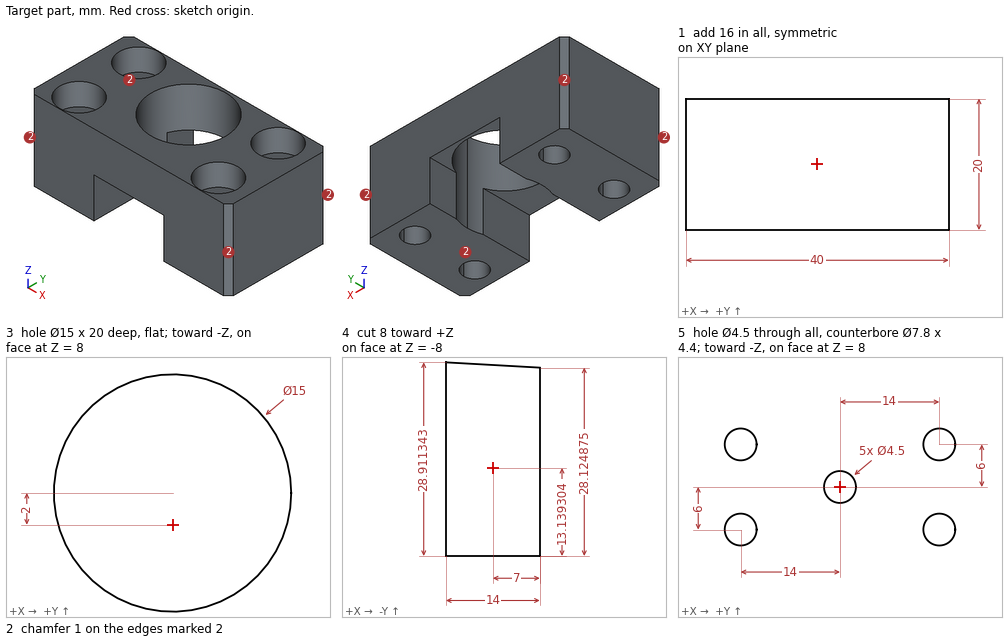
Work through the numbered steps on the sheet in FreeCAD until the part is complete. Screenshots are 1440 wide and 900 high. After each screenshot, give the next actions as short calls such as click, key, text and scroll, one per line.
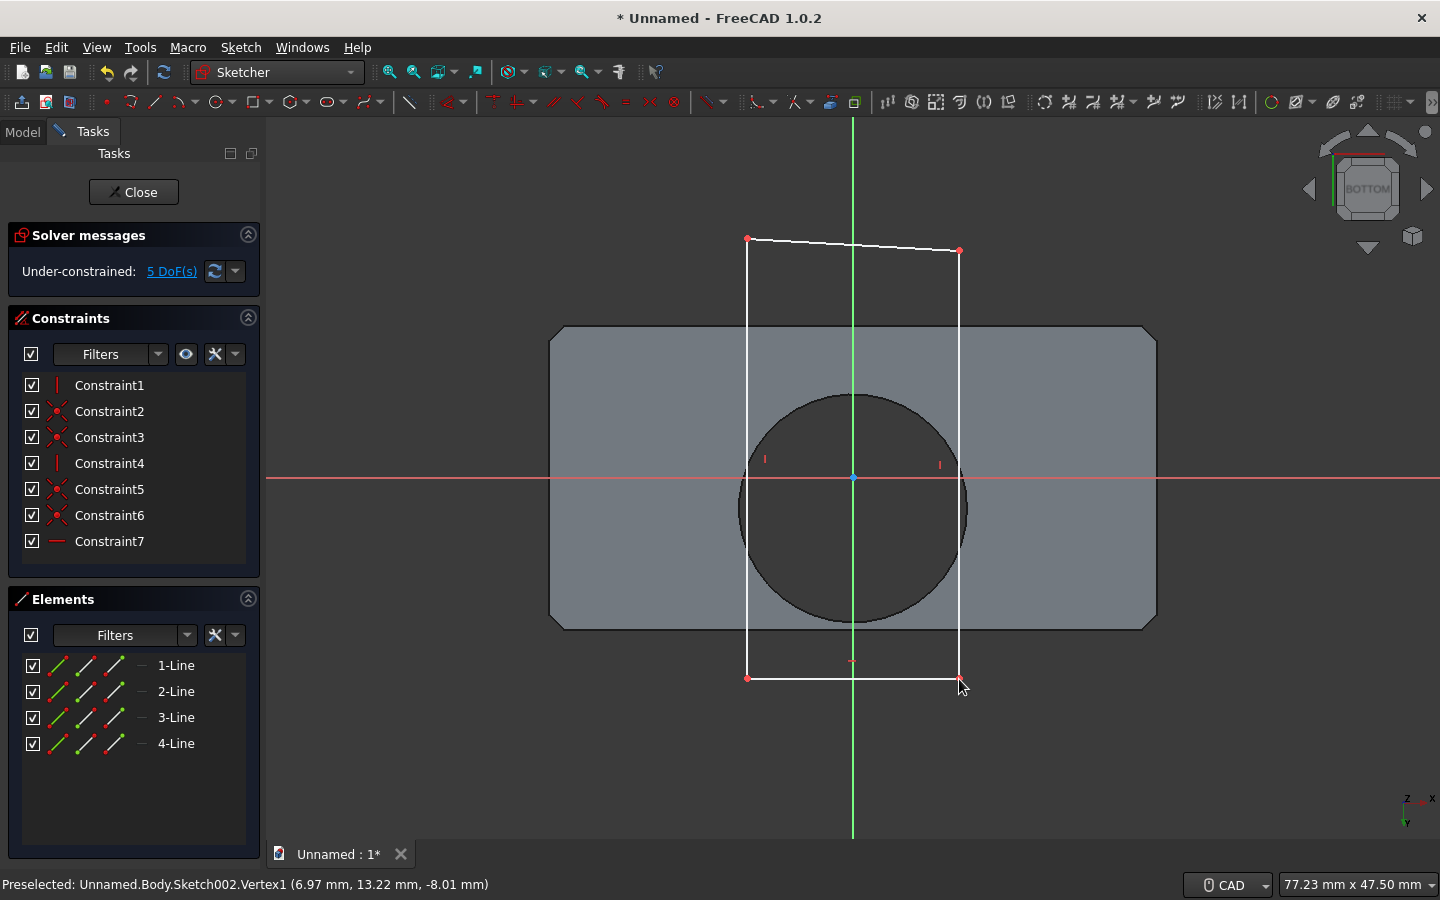
key(d)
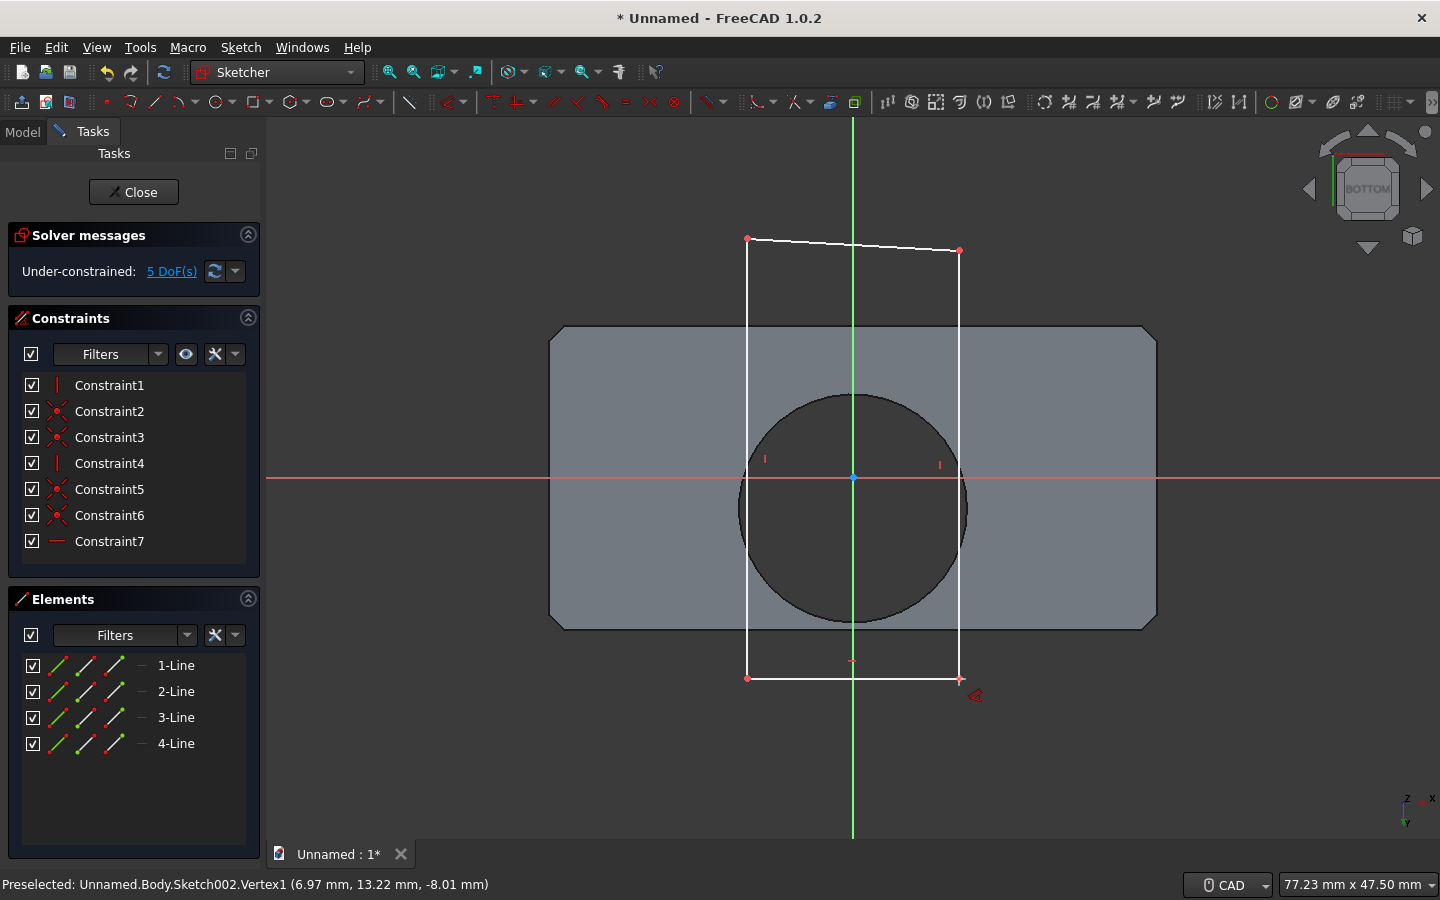
click(811, 679)
click(804, 713)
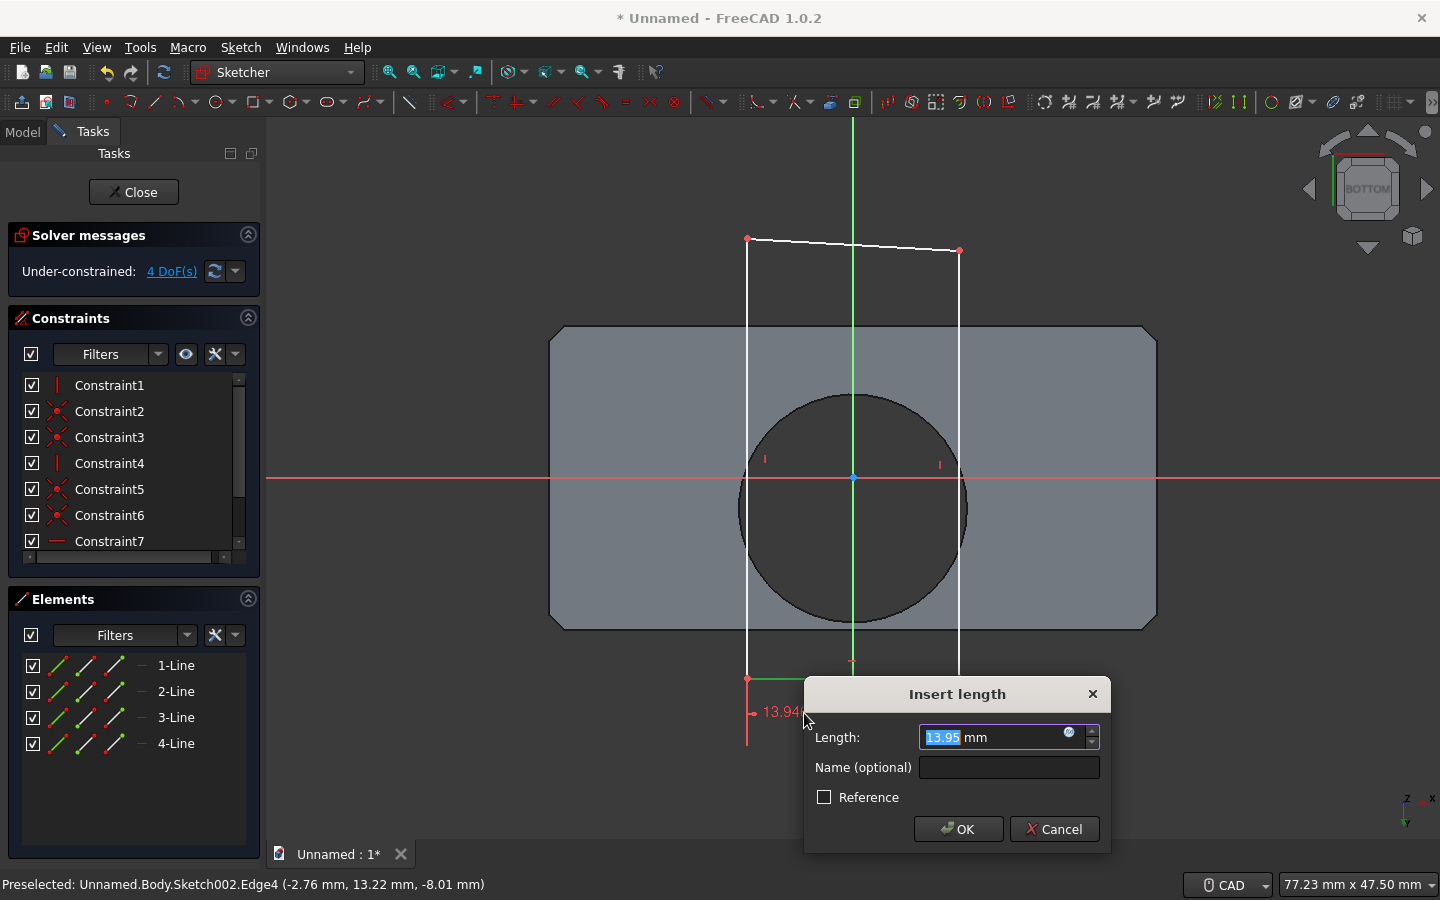
text(14)
key(Return)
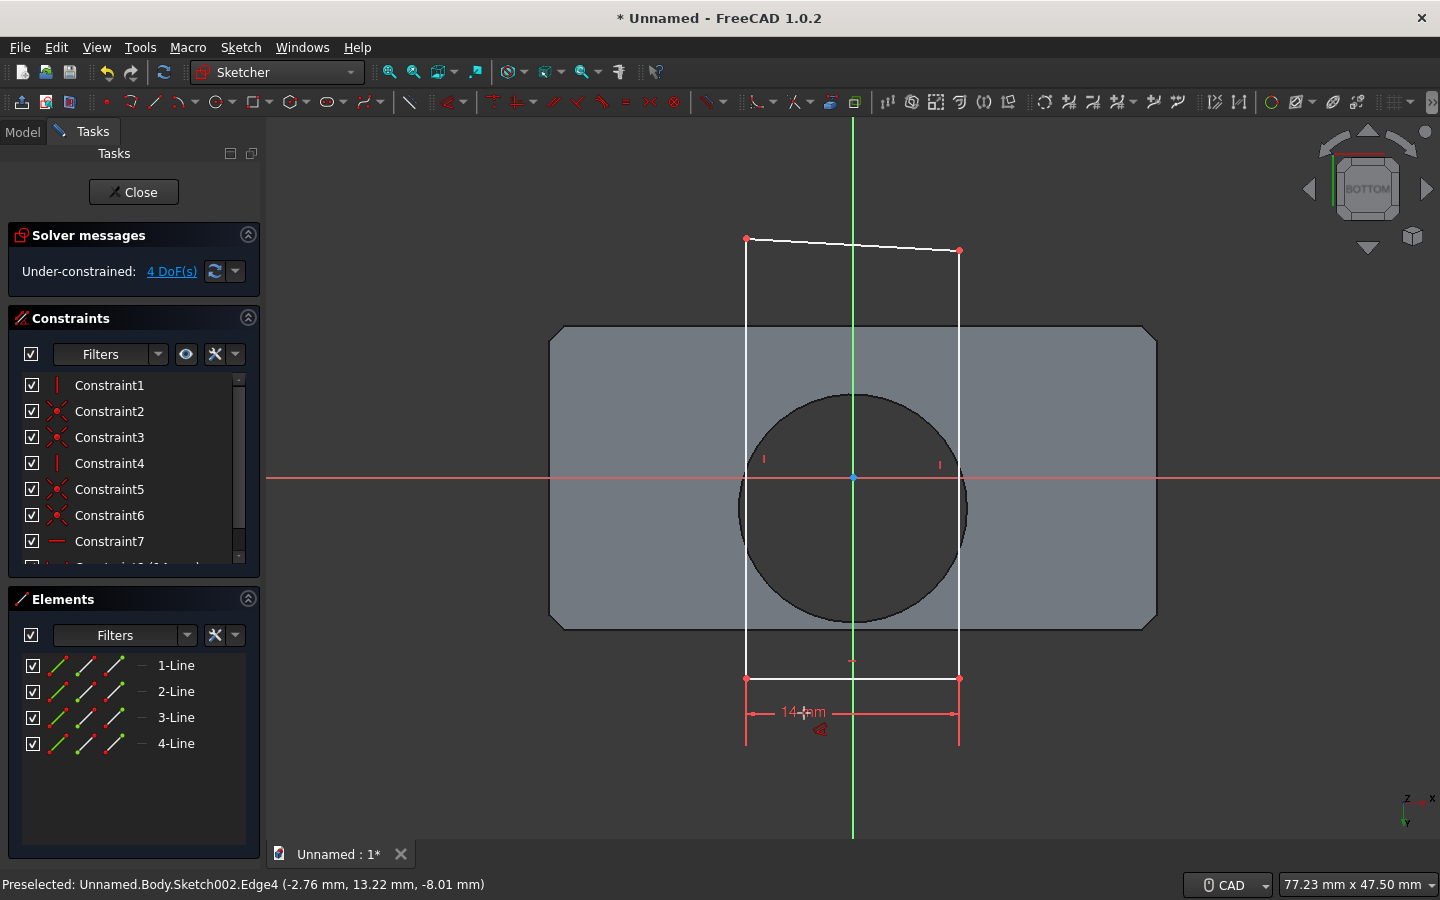
click(959, 679)
click(906, 713)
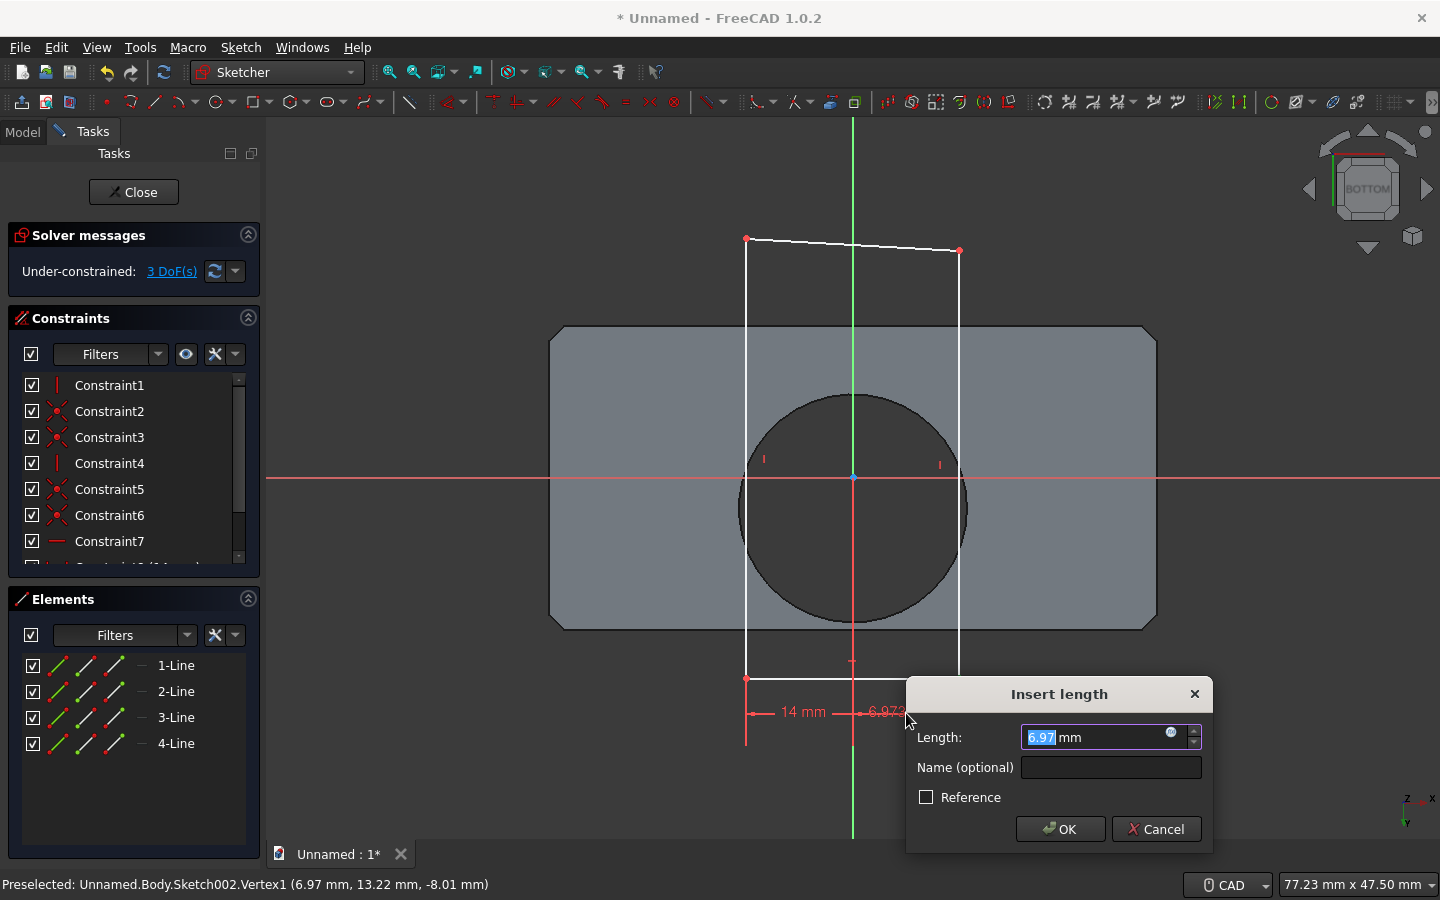
text(7)
key(Return)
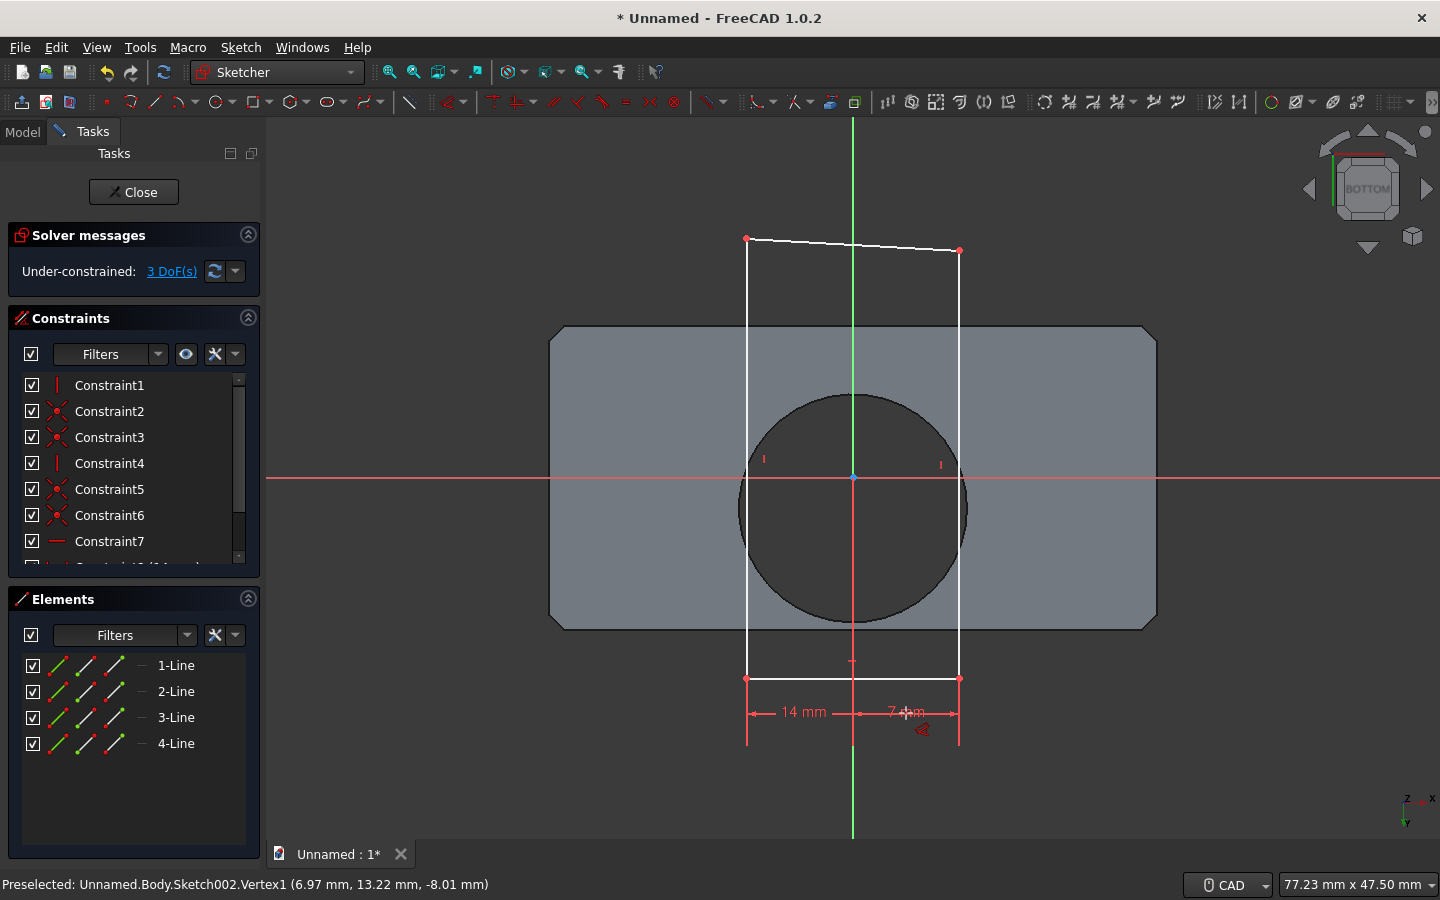
click(959, 551)
click(993, 465)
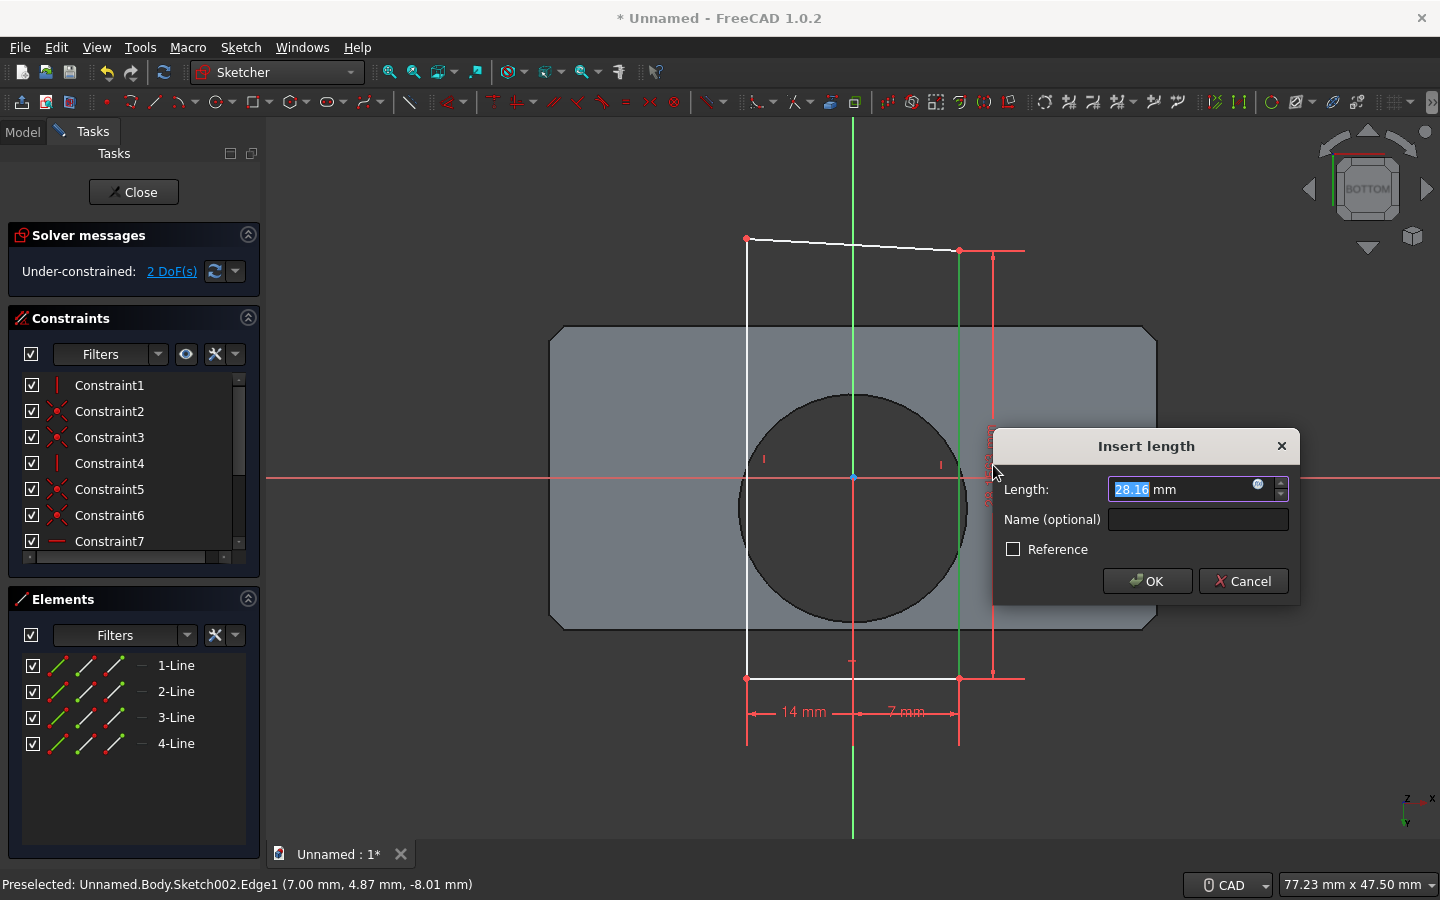
text(28.124875)
key(Return)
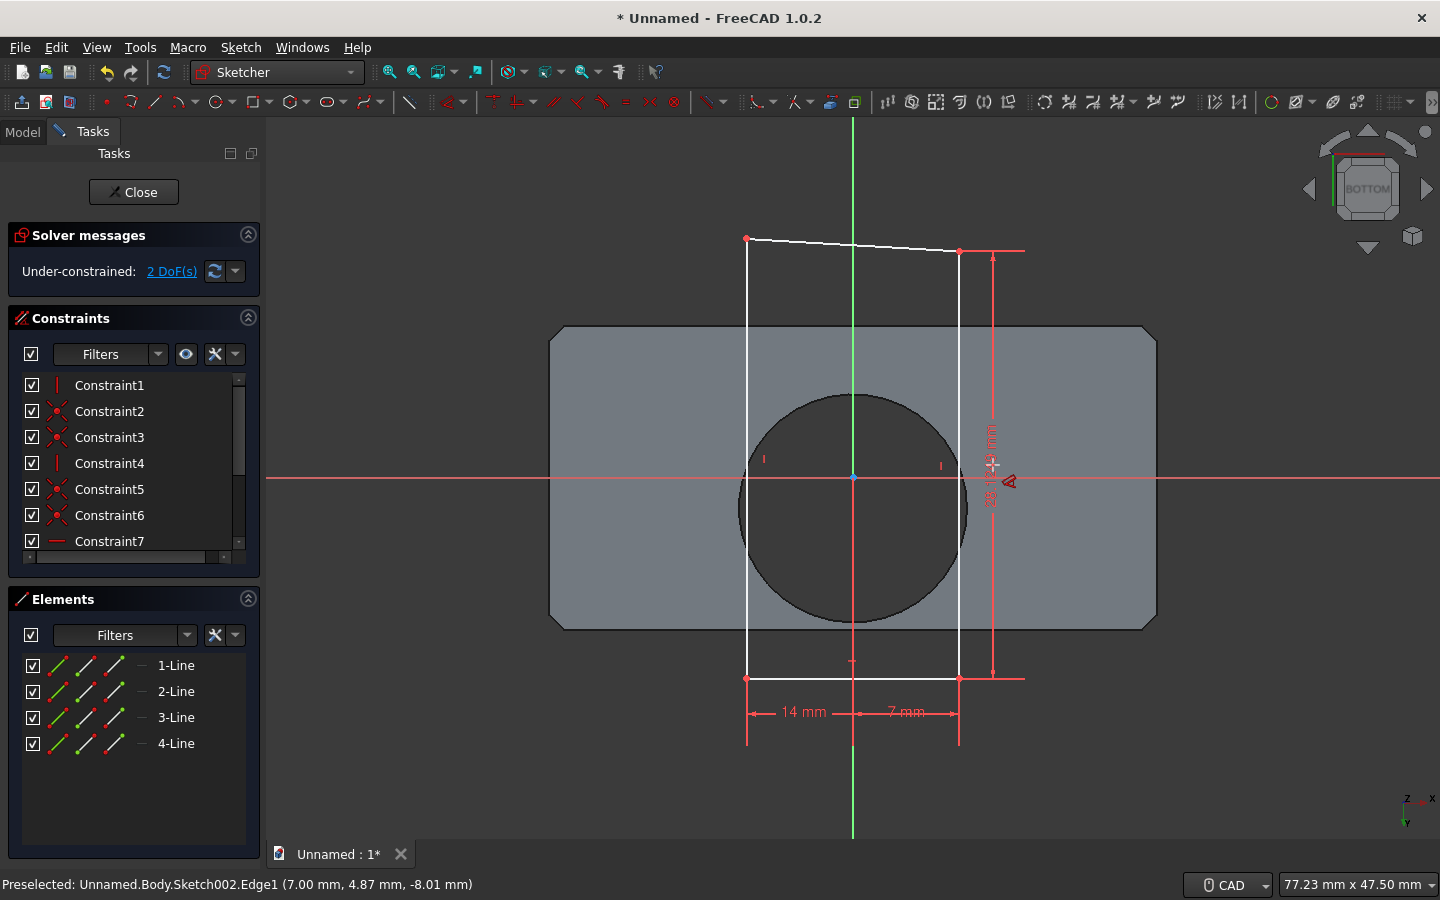
click(747, 371)
click(713, 459)